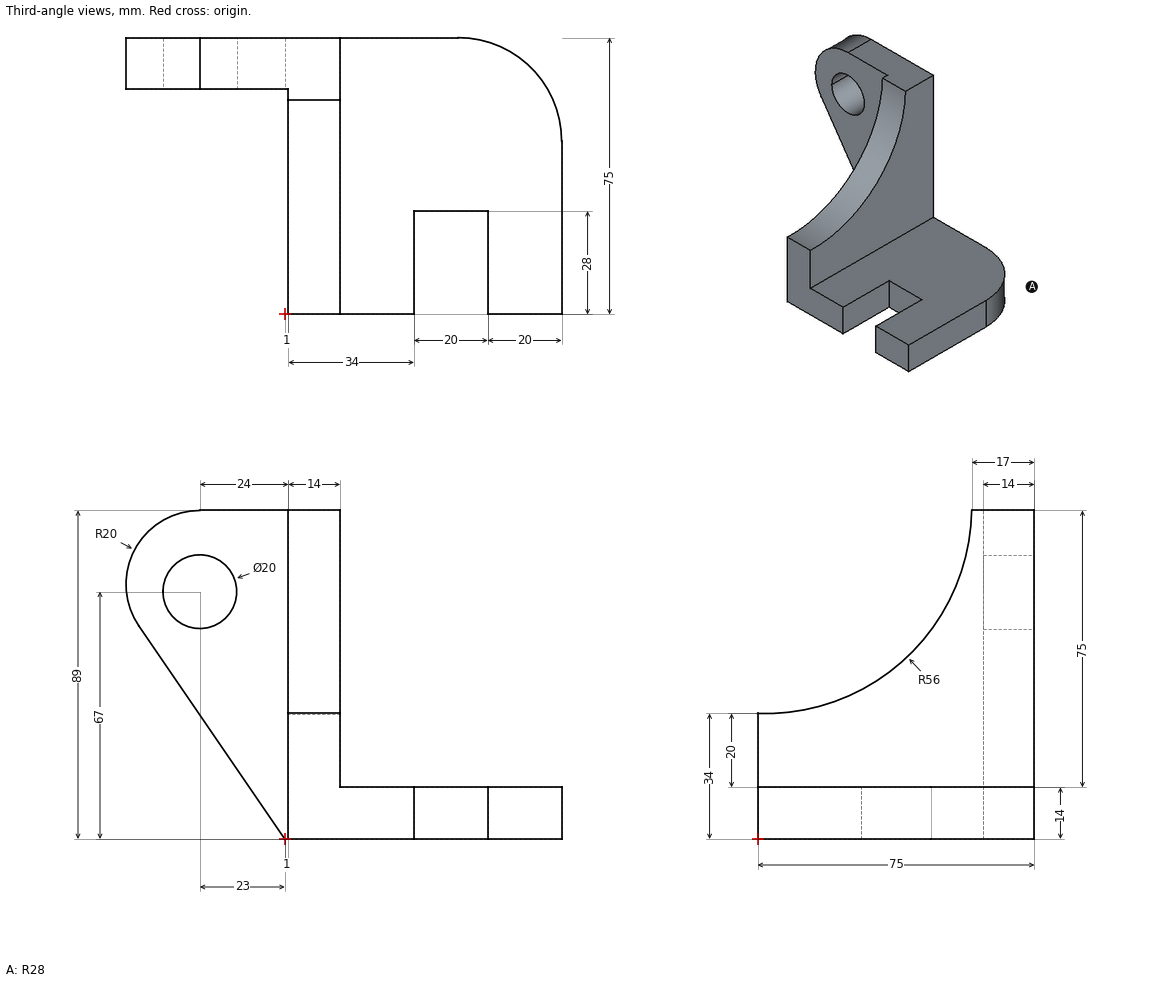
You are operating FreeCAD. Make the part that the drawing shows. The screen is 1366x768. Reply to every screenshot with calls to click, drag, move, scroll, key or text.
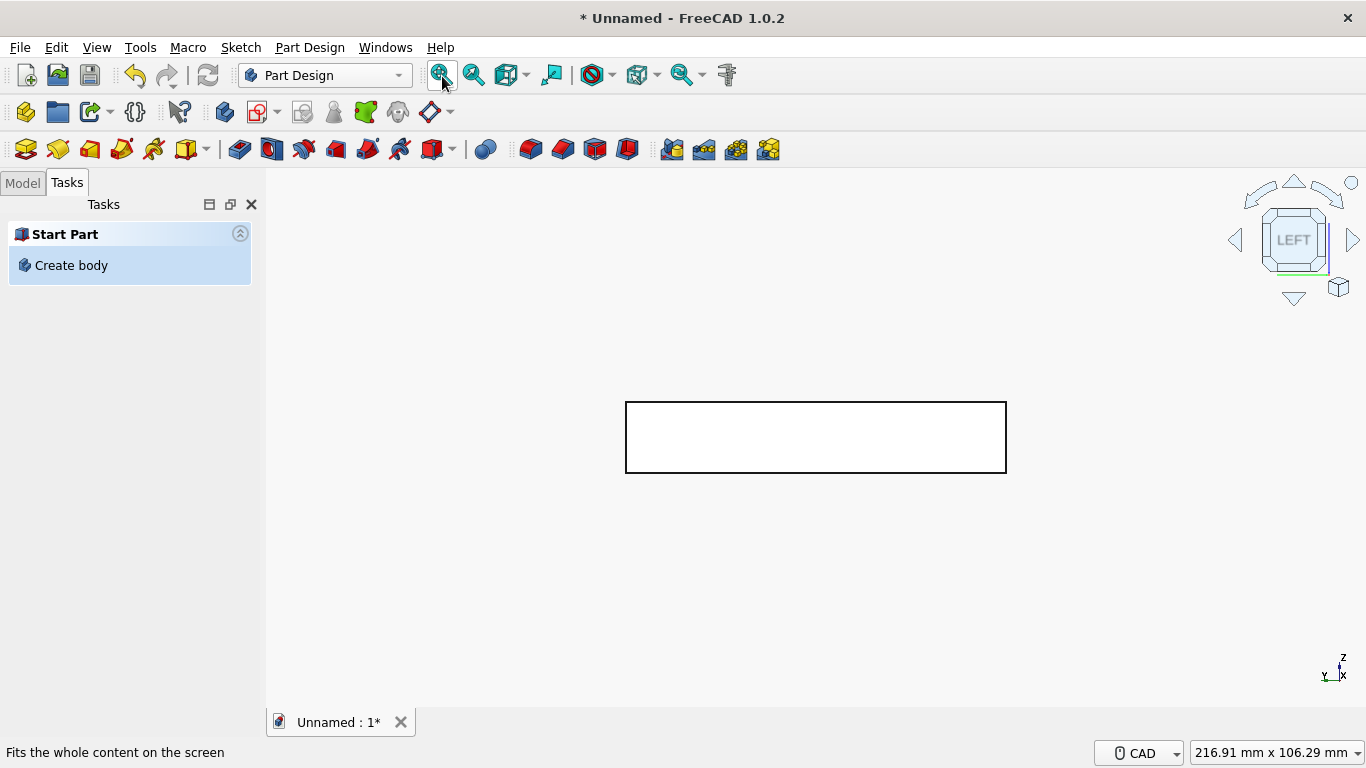
click(707, 436)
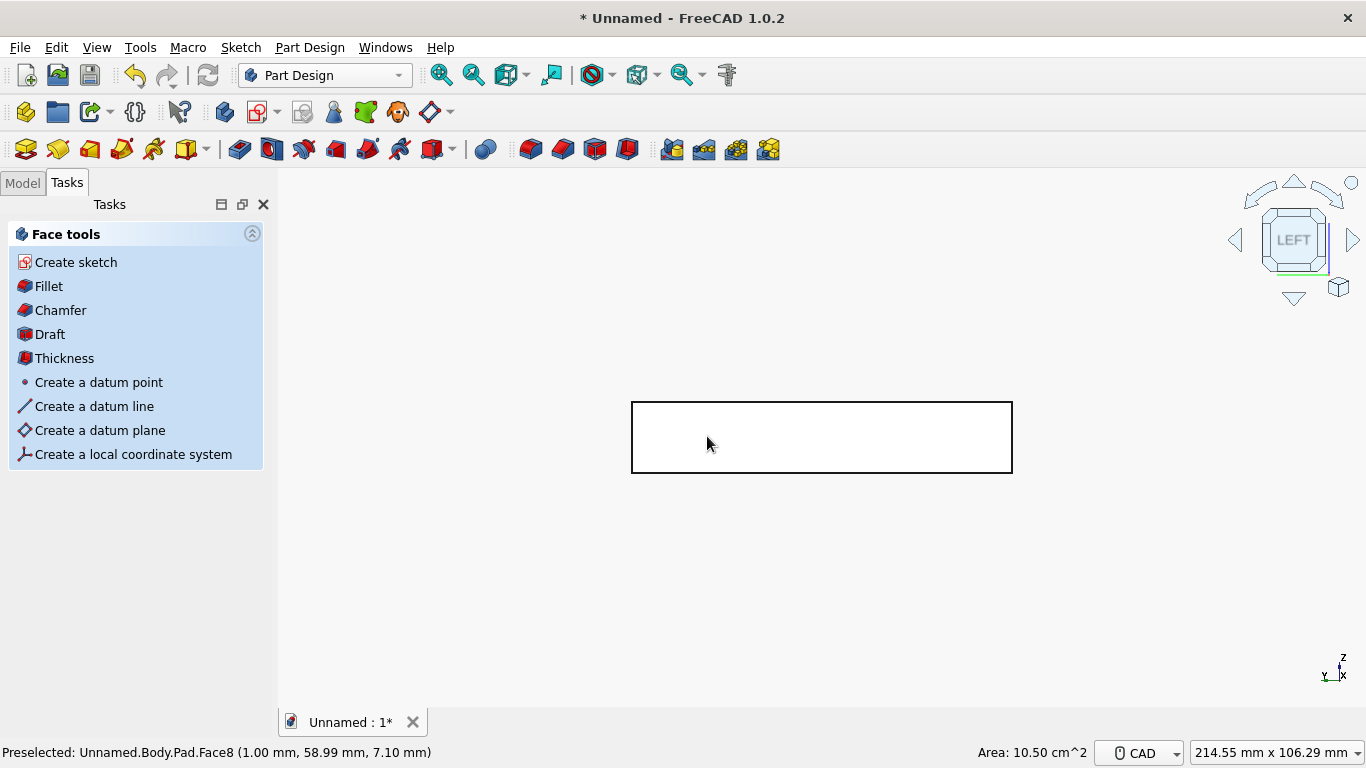
click(258, 112)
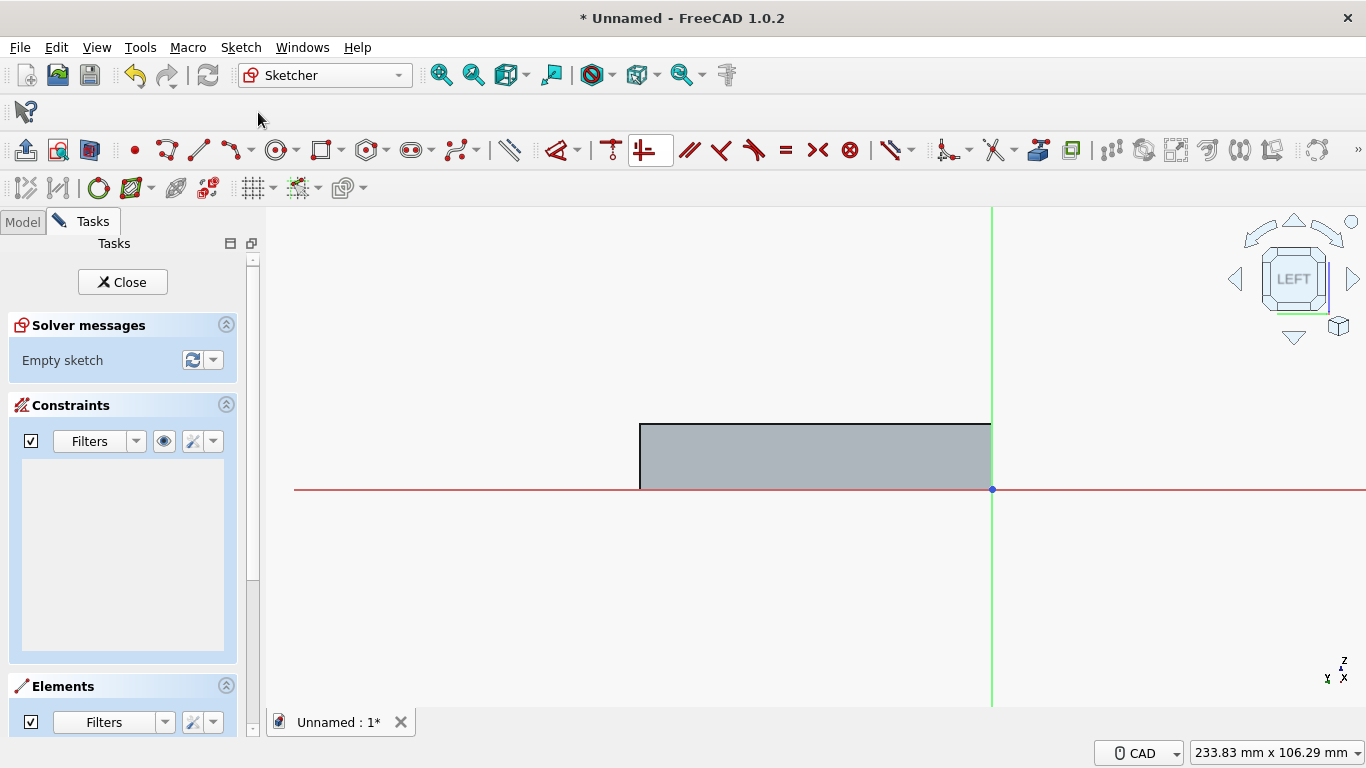
scroll(608, 679, down, 2)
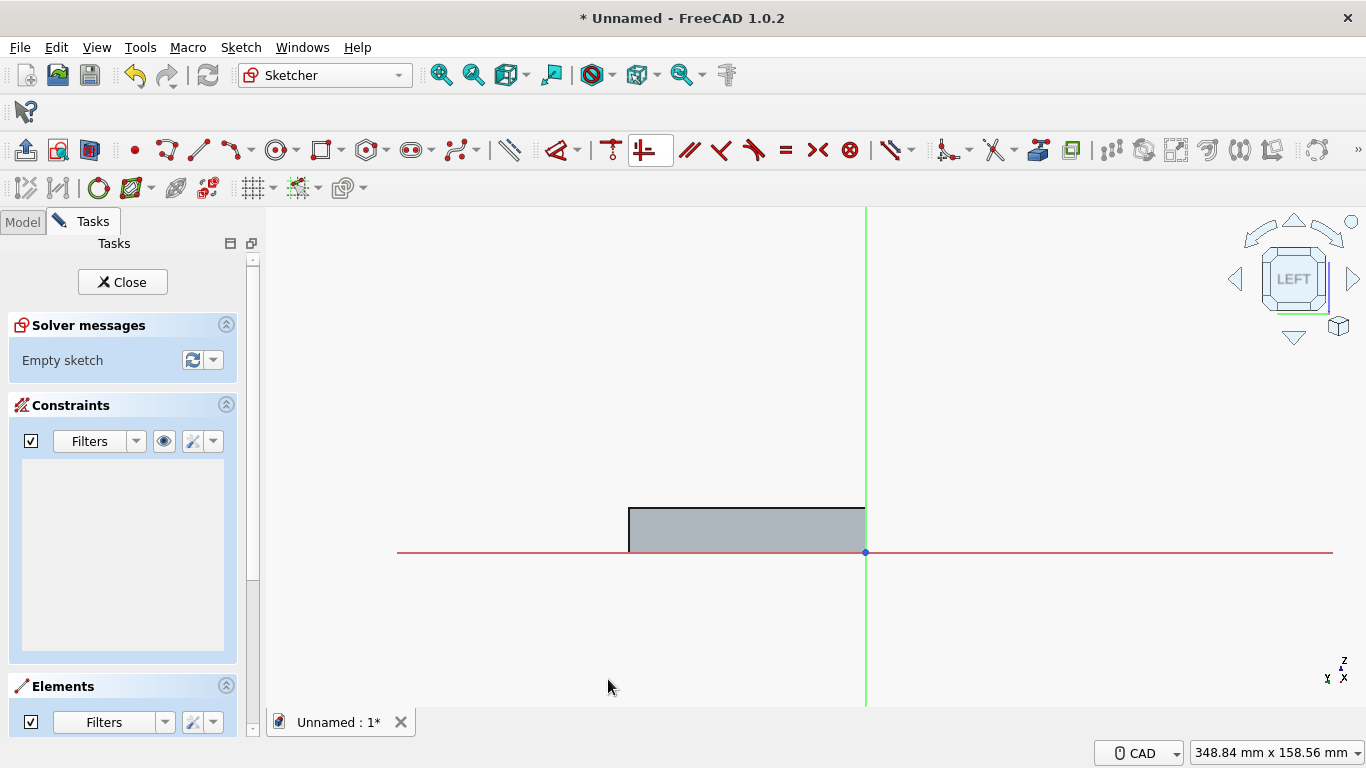
click(168, 150)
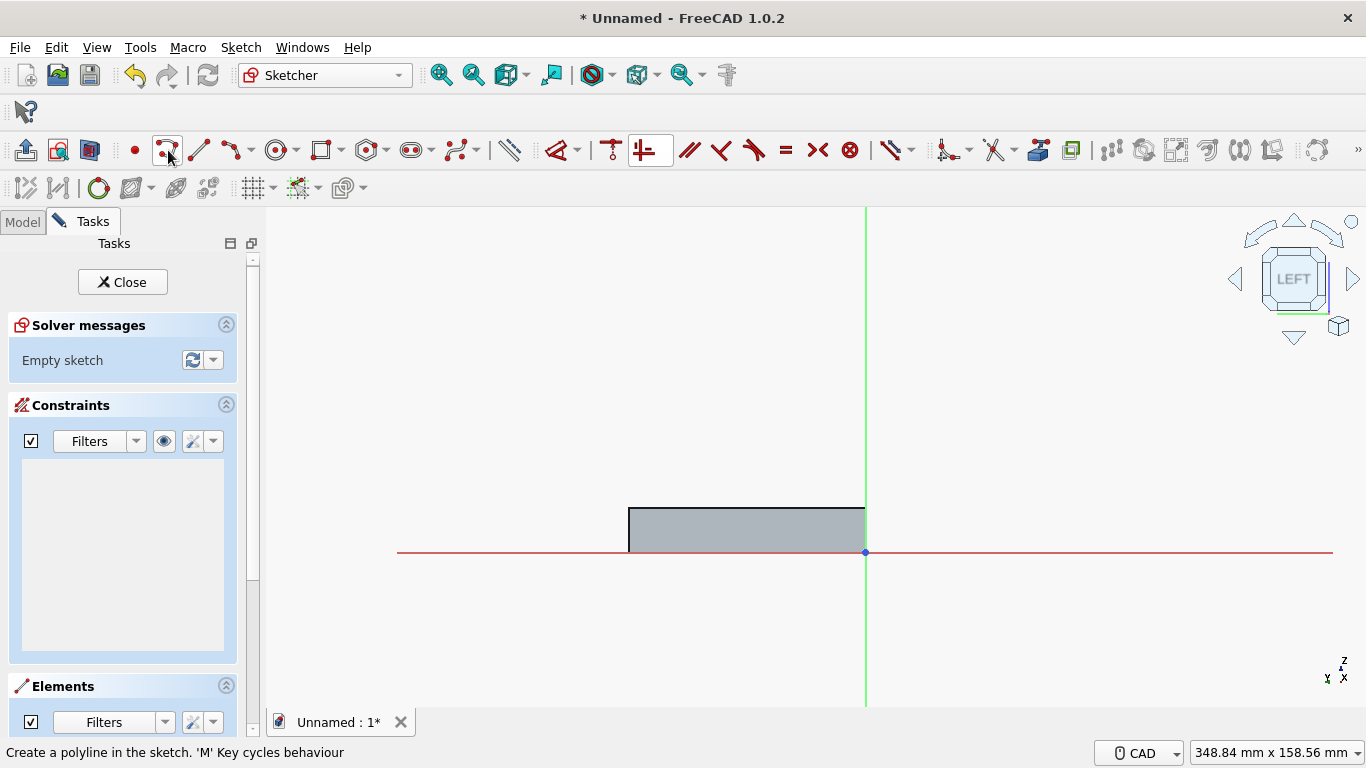
click(866, 445)
click(857, 508)
click(629, 508)
click(629, 272)
click(683, 272)
right_click(683, 272)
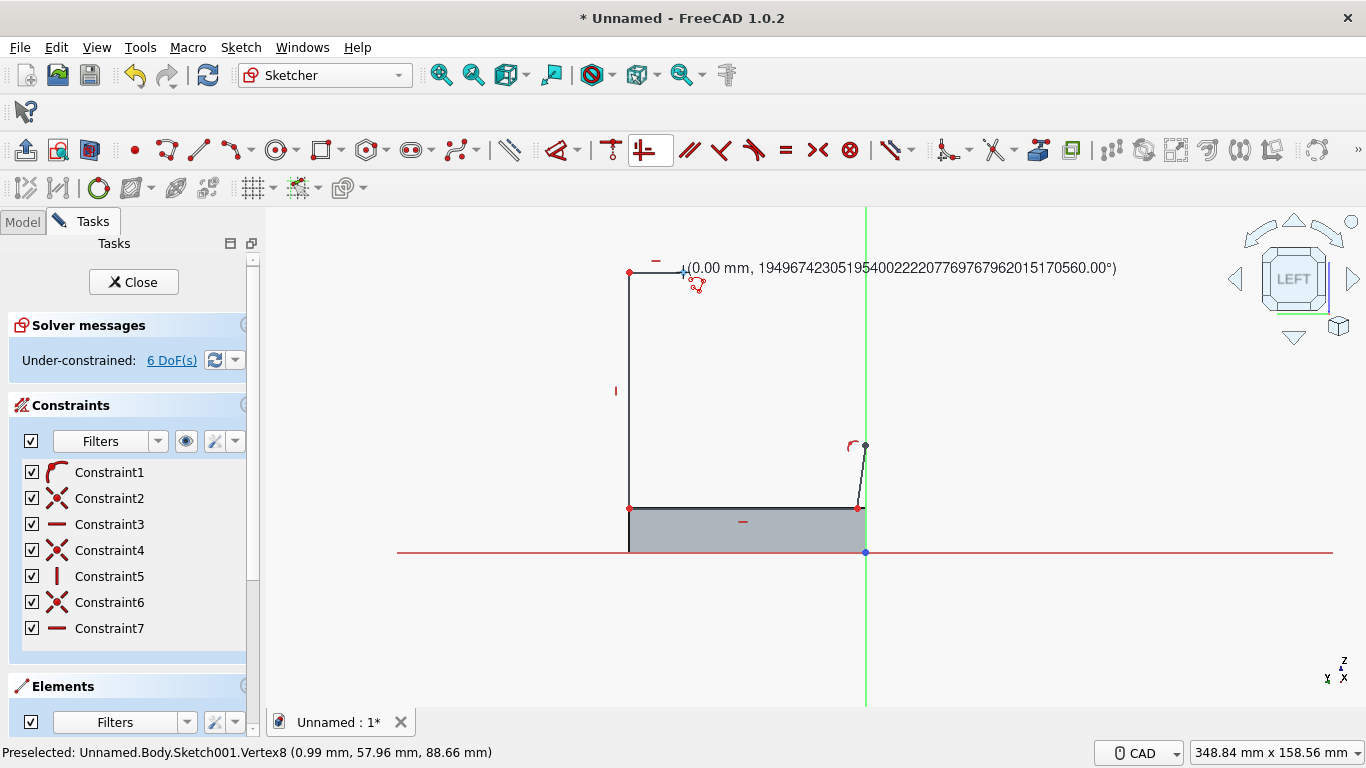
click(232, 150)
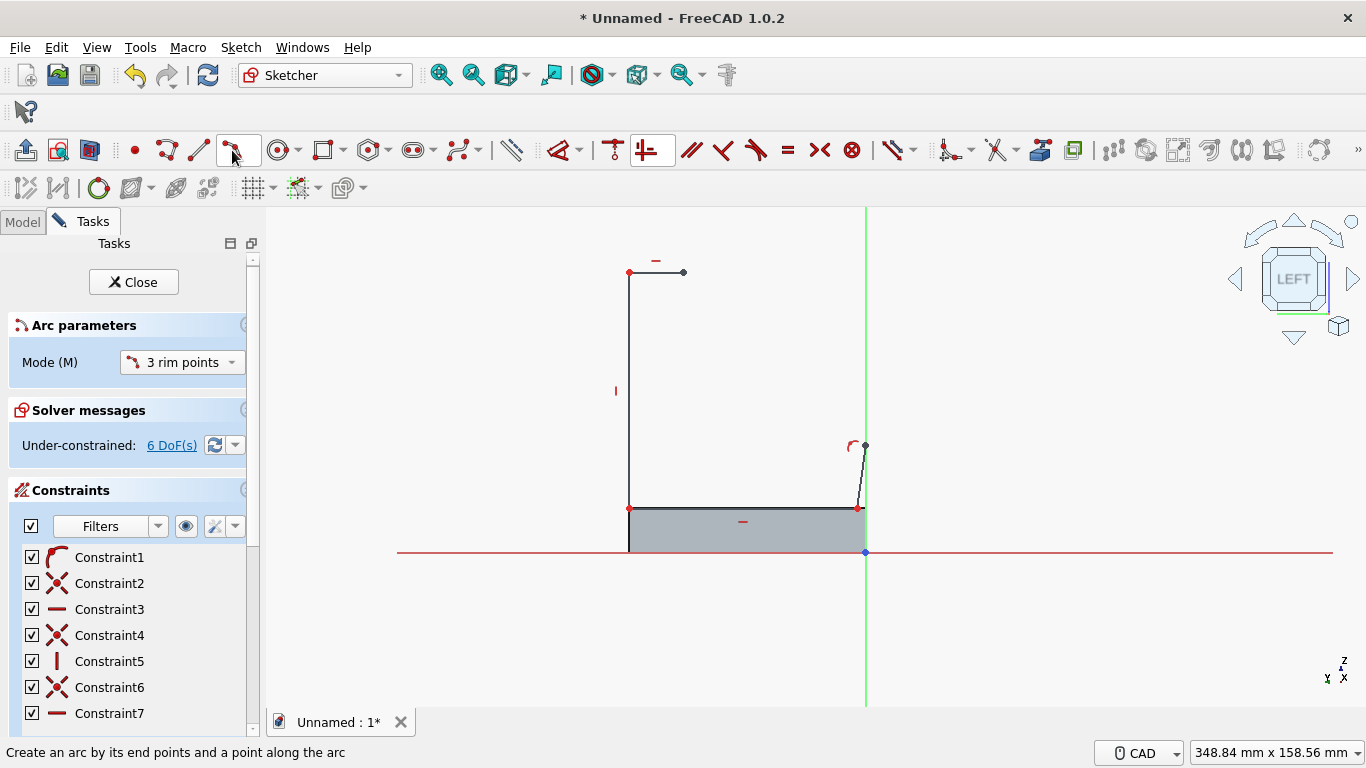
click(683, 273)
click(866, 446)
click(738, 397)
key(Escape)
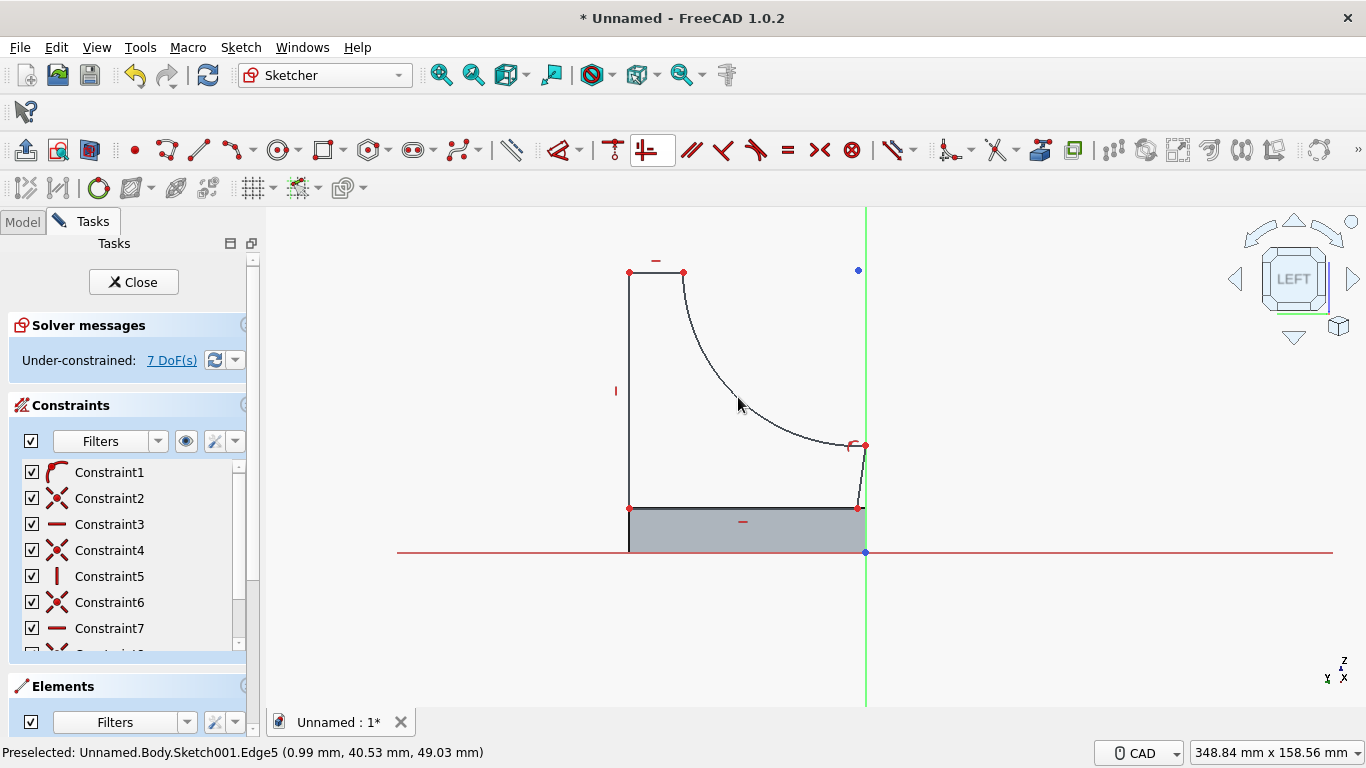
click(863, 465)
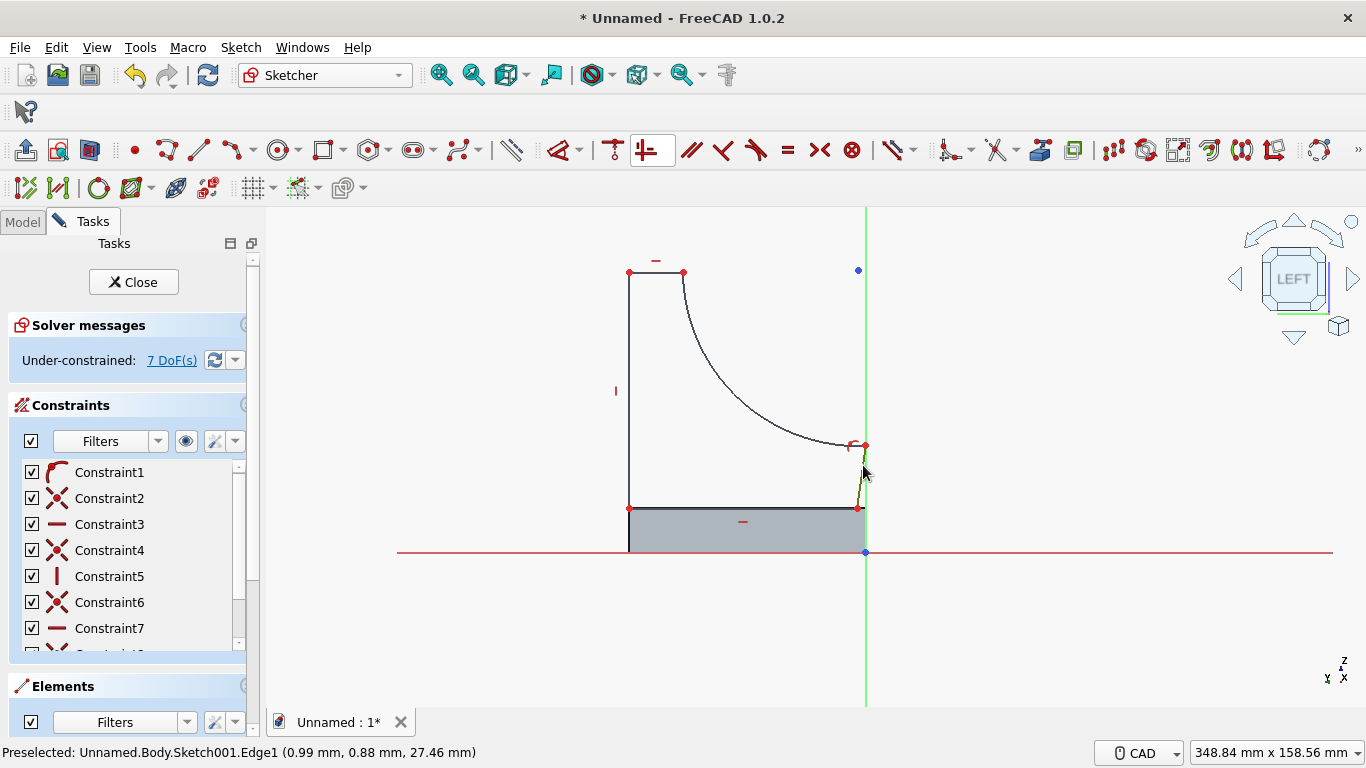
key(v)